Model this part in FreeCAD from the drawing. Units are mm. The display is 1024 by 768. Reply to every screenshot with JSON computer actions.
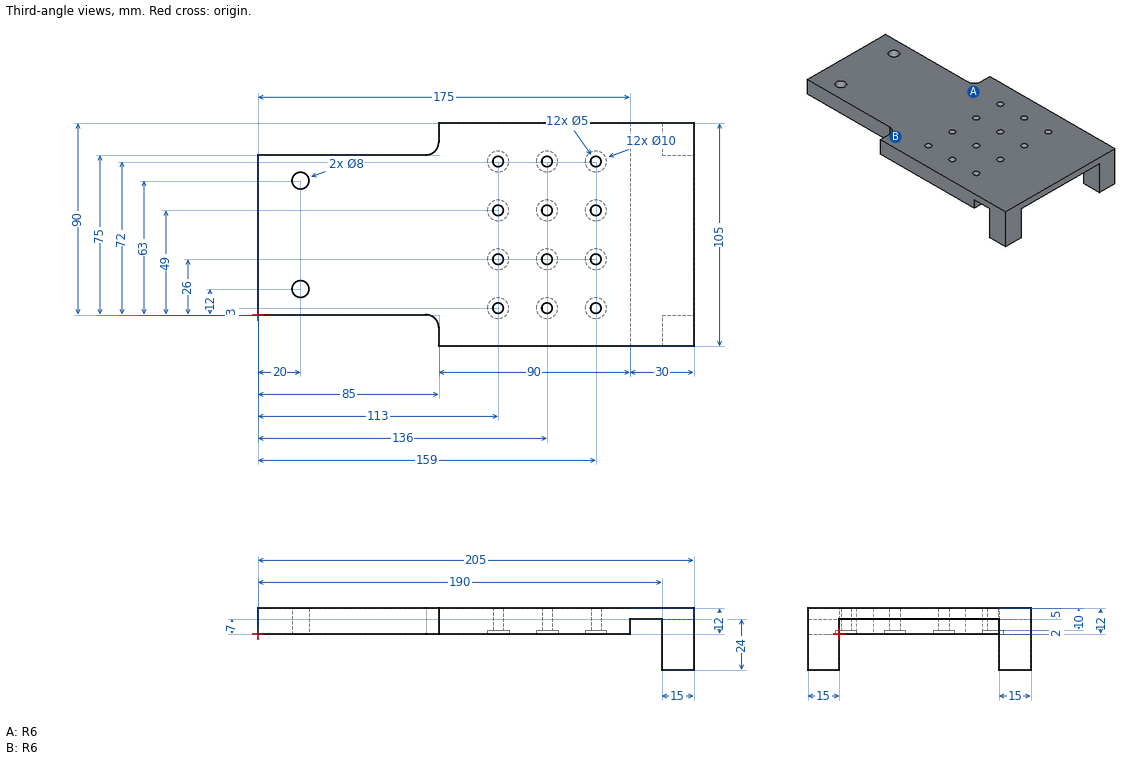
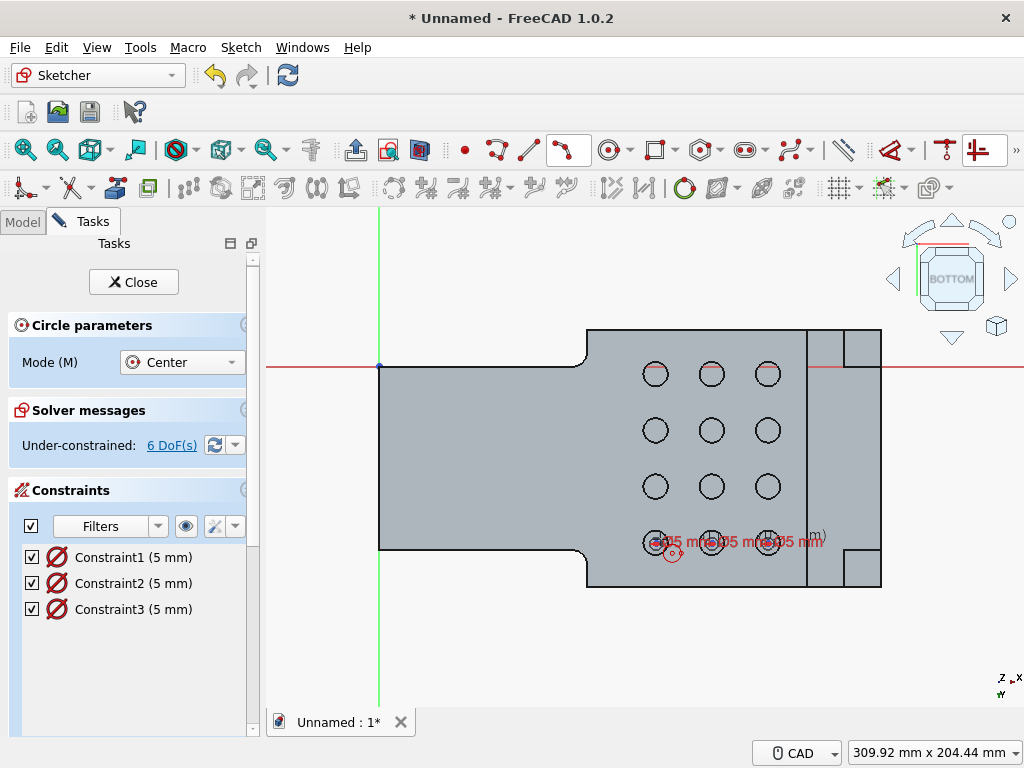
{"action": "scroll", "coordinate": [656, 487], "scroll_direction": "up", "scroll_amount": 7}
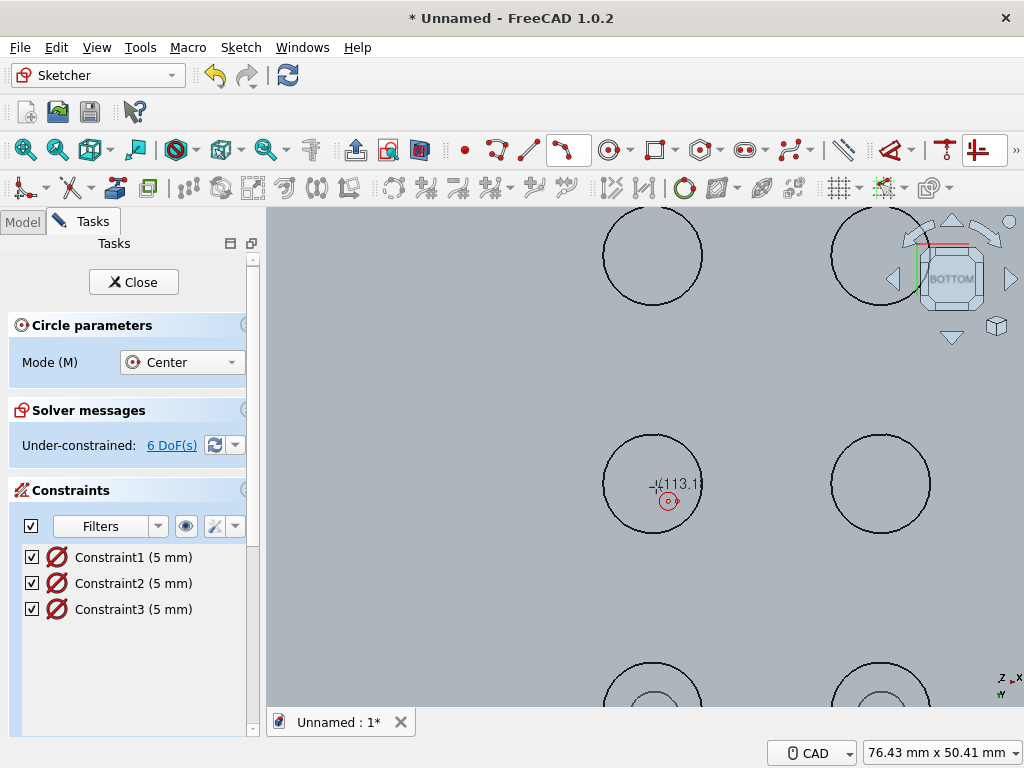
{"action": "scroll", "coordinate": [656, 486], "scroll_direction": "down", "scroll_amount": 7}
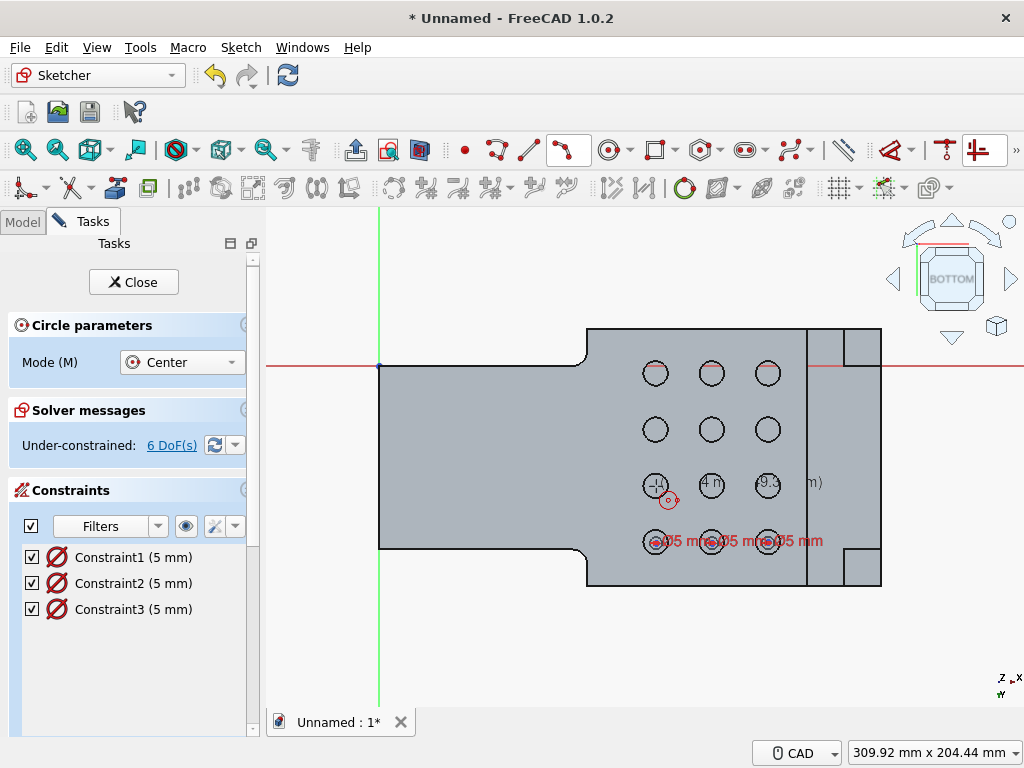
{"action": "left_click", "coordinate": [656, 486]}
{"action": "mouse_move", "coordinate": [660, 482]}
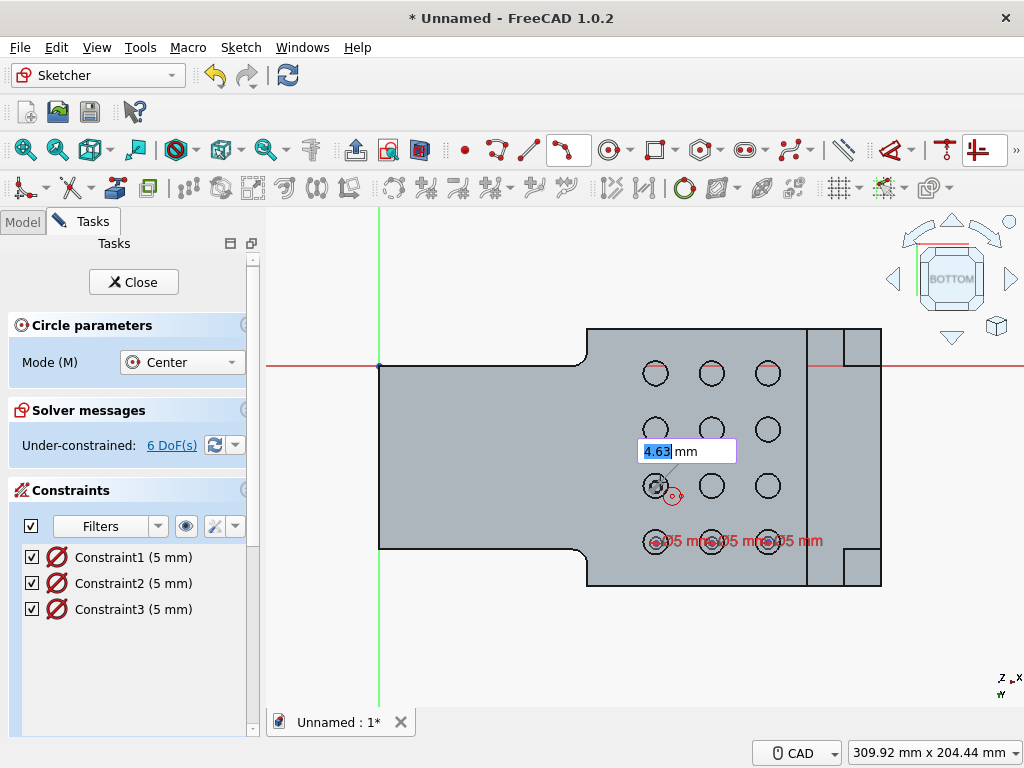
{"action": "type", "text": "5"}
{"action": "key", "text": "Return"}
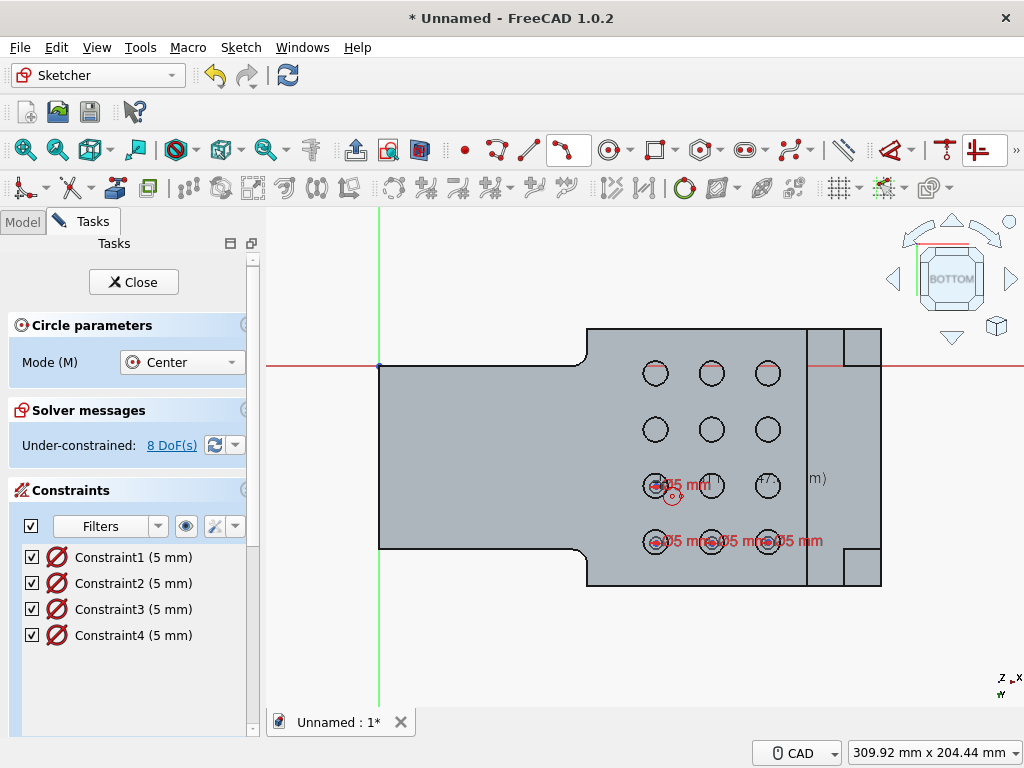
{"action": "scroll", "coordinate": [712, 486], "scroll_direction": "up", "scroll_amount": 7}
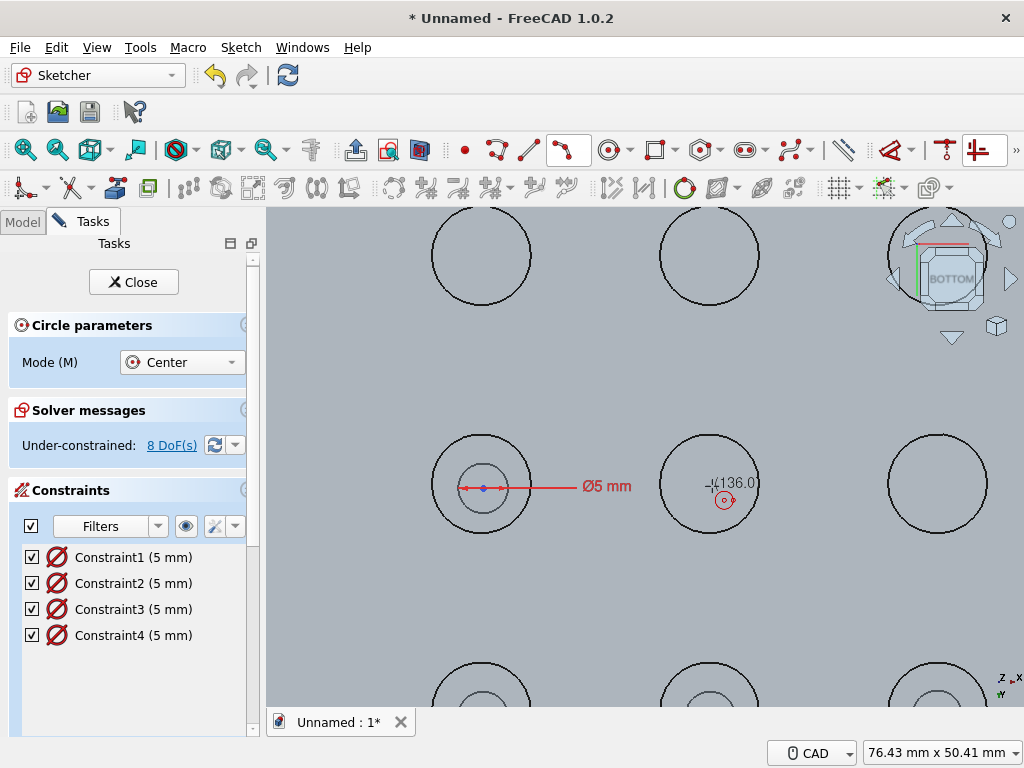
{"action": "scroll", "coordinate": [712, 486], "scroll_direction": "down", "scroll_amount": 7}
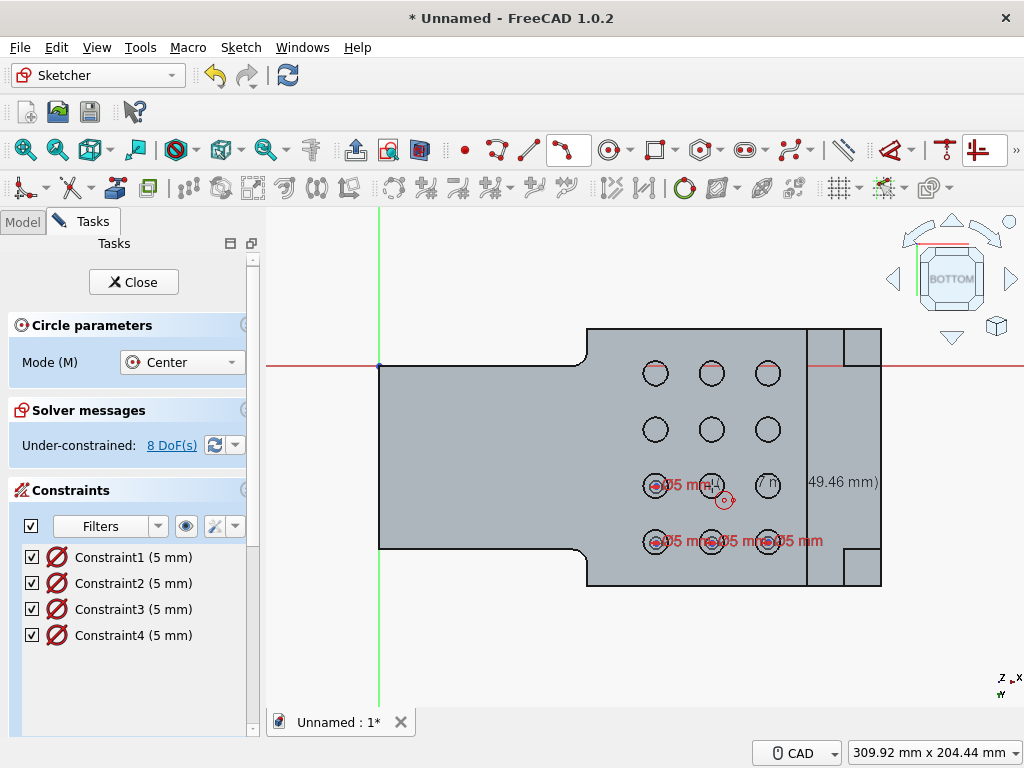
{"action": "left_click", "coordinate": [712, 486]}
{"action": "mouse_move", "coordinate": [716, 482]}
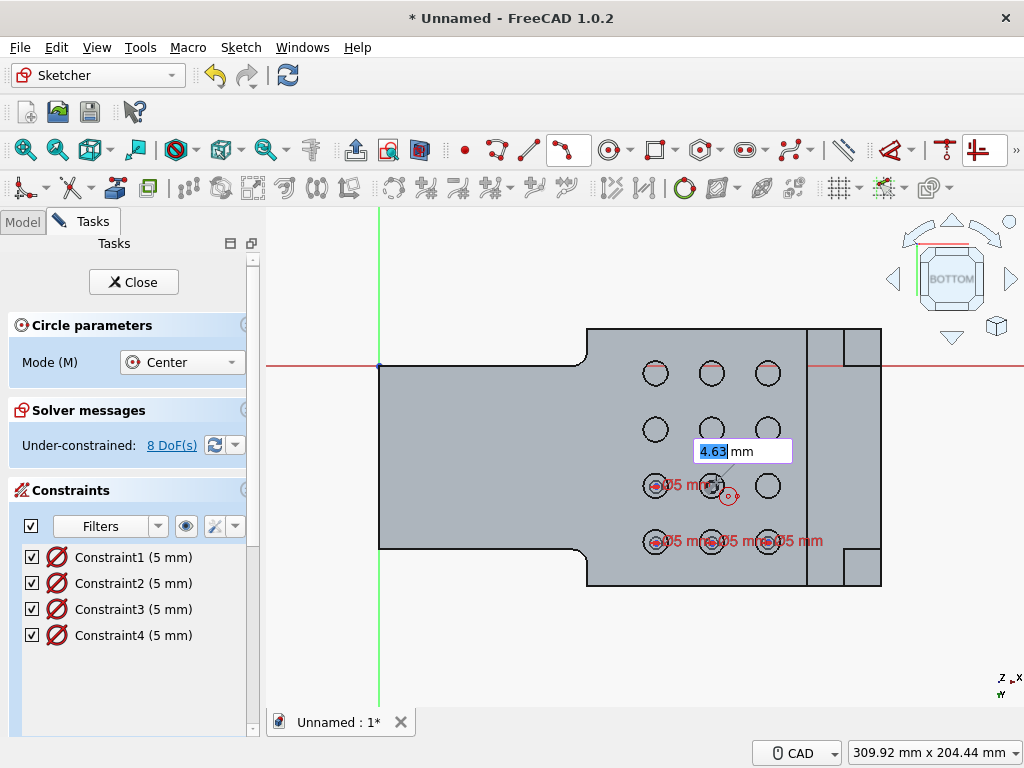
{"action": "type", "text": "5"}
{"action": "key", "text": "Return"}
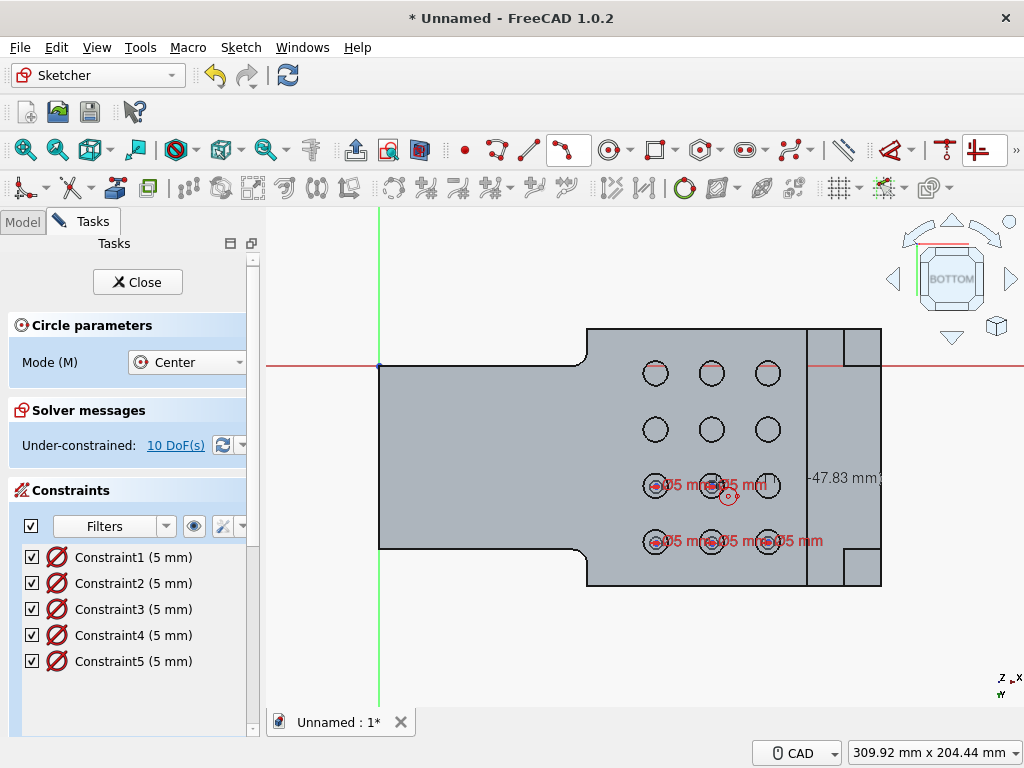
{"action": "scroll", "coordinate": [768, 486], "scroll_direction": "up", "scroll_amount": 7}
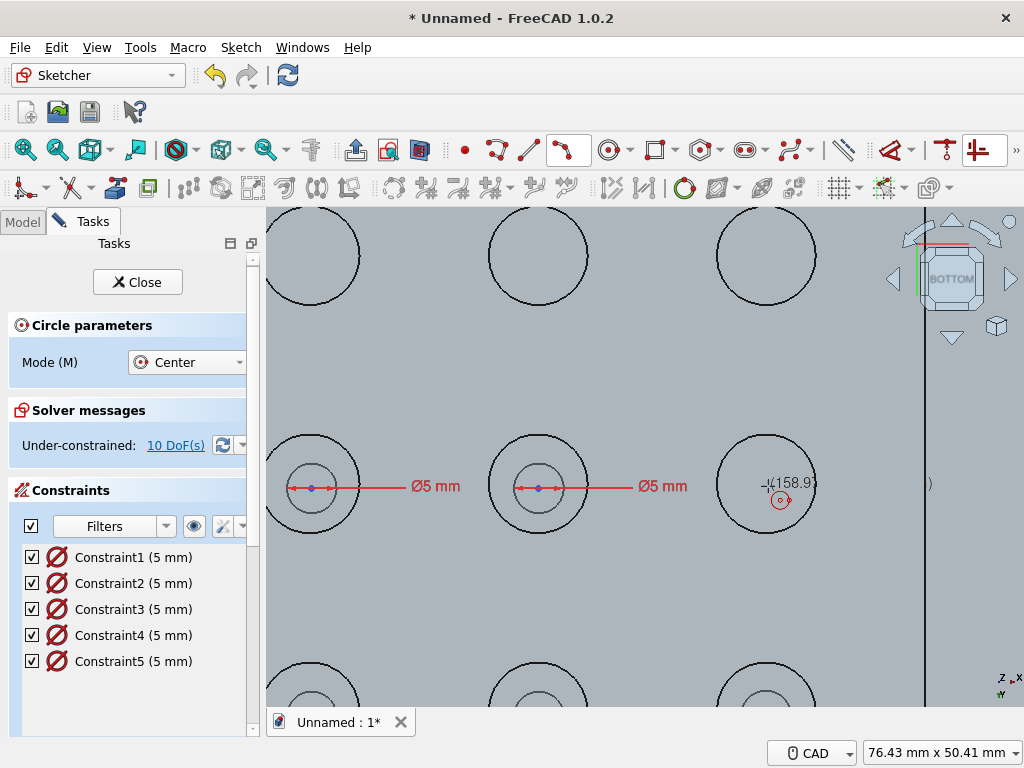
{"action": "scroll", "coordinate": [768, 486], "scroll_direction": "down", "scroll_amount": 7}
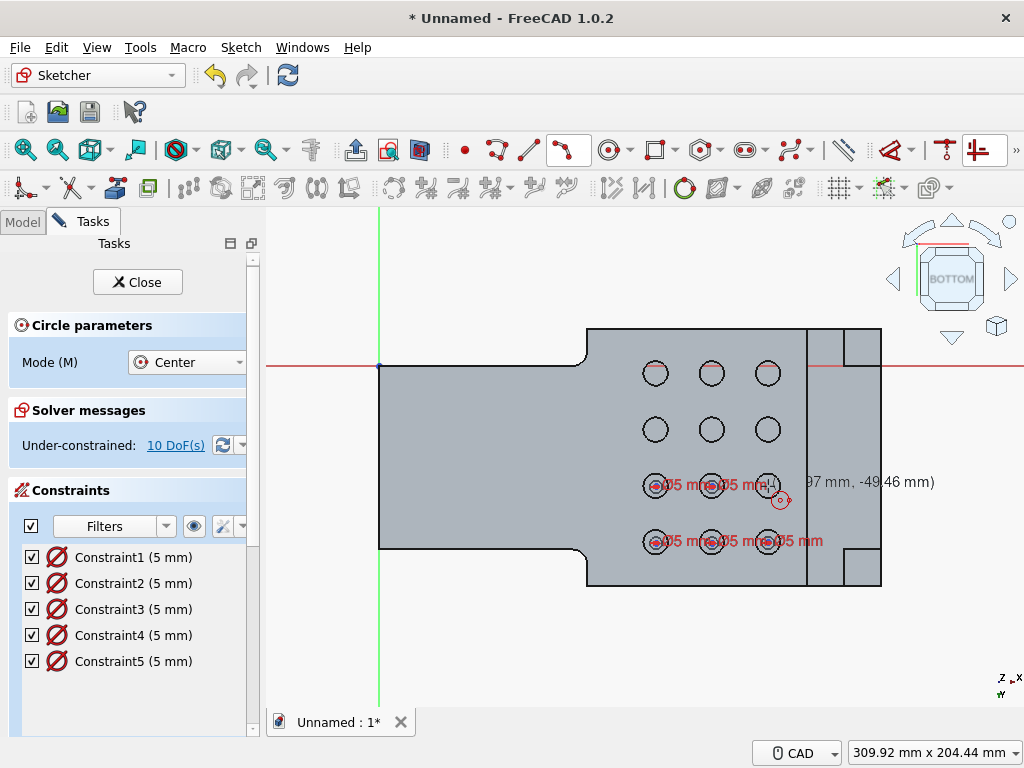
{"action": "left_click", "coordinate": [768, 486]}
{"action": "mouse_move", "coordinate": [772, 482]}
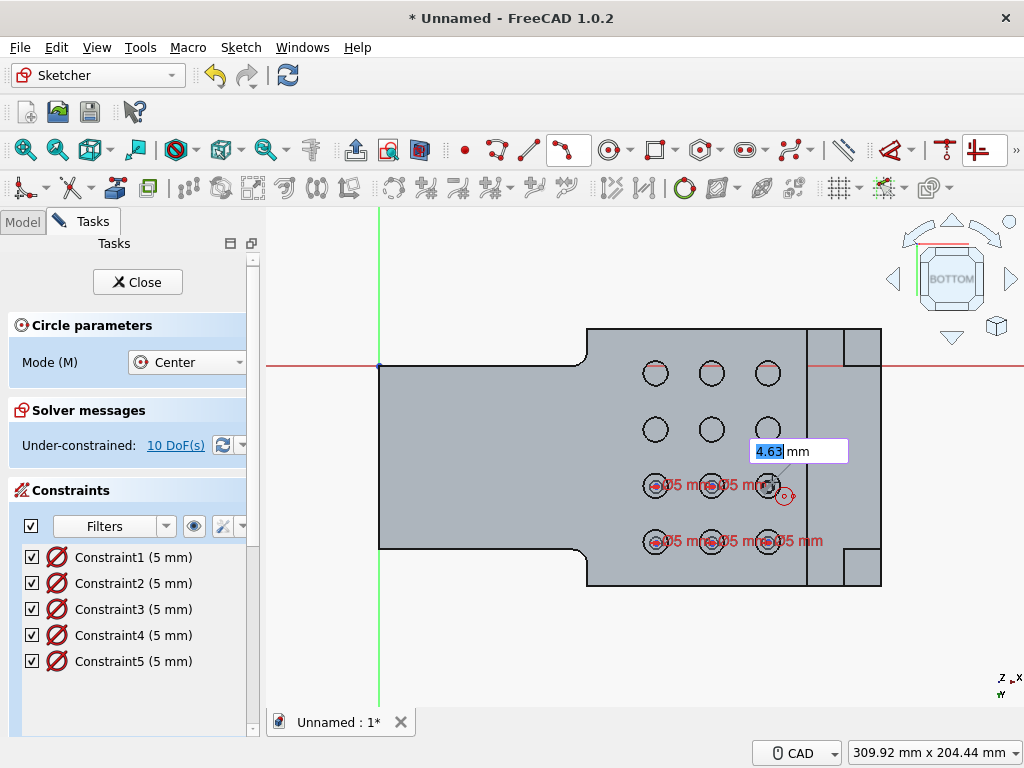
{"action": "type", "text": "5"}
{"action": "key", "text": "Return"}